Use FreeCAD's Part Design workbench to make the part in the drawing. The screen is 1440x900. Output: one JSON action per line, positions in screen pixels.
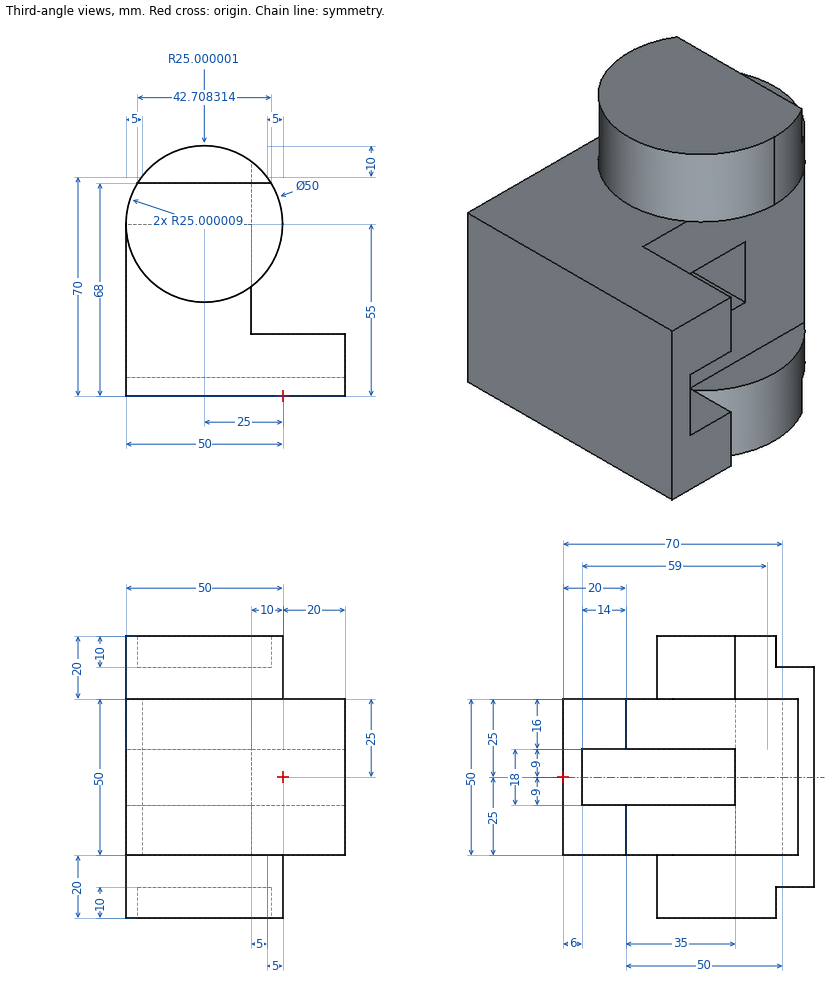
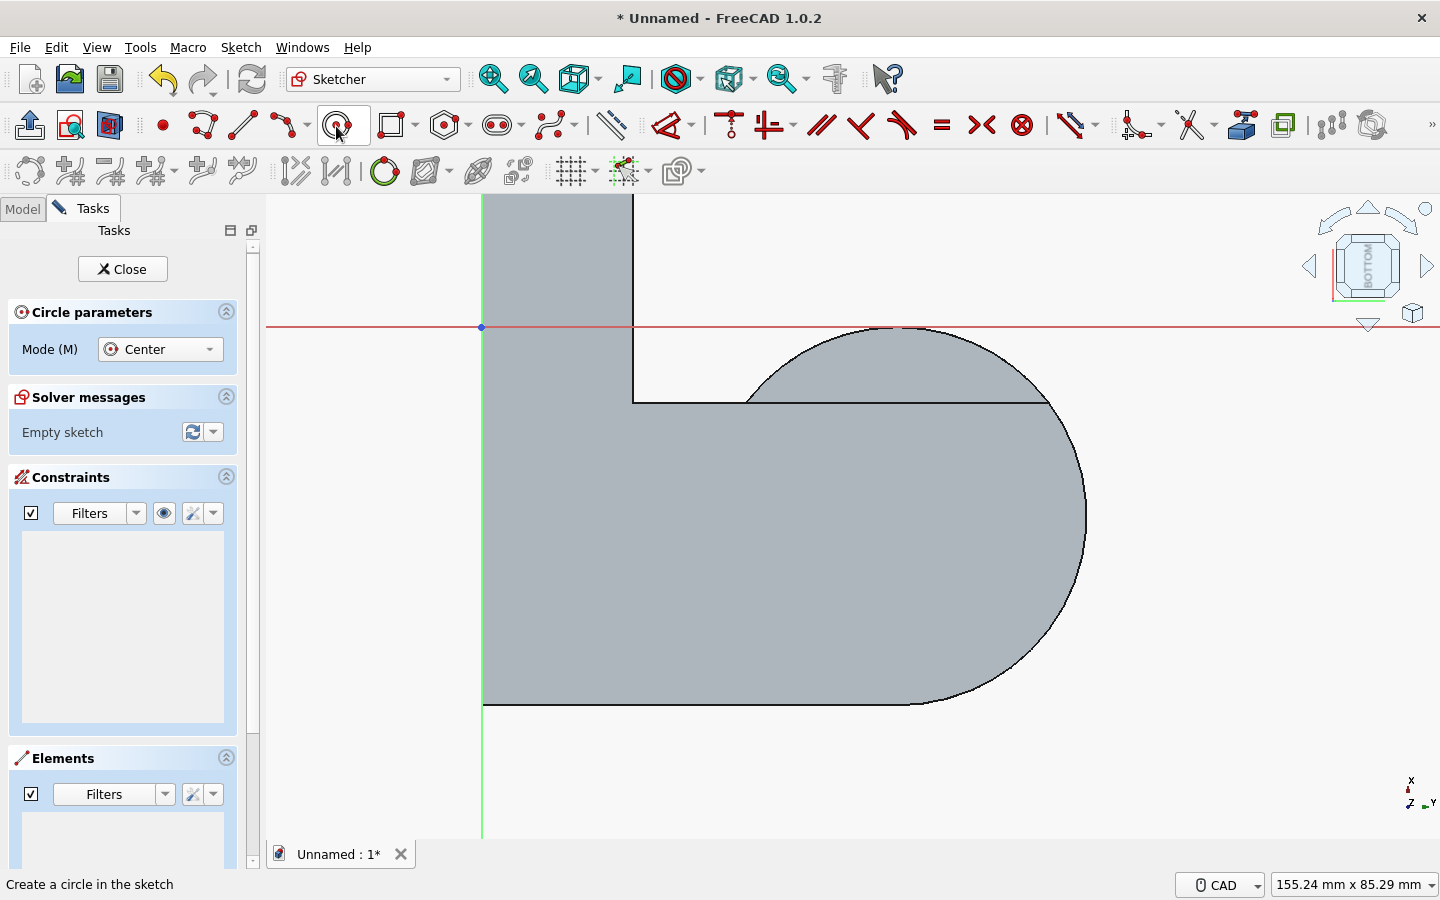
{"action": "left_click", "coordinate": [898, 516]}
{"action": "mouse_move", "coordinate": [1031, 383]}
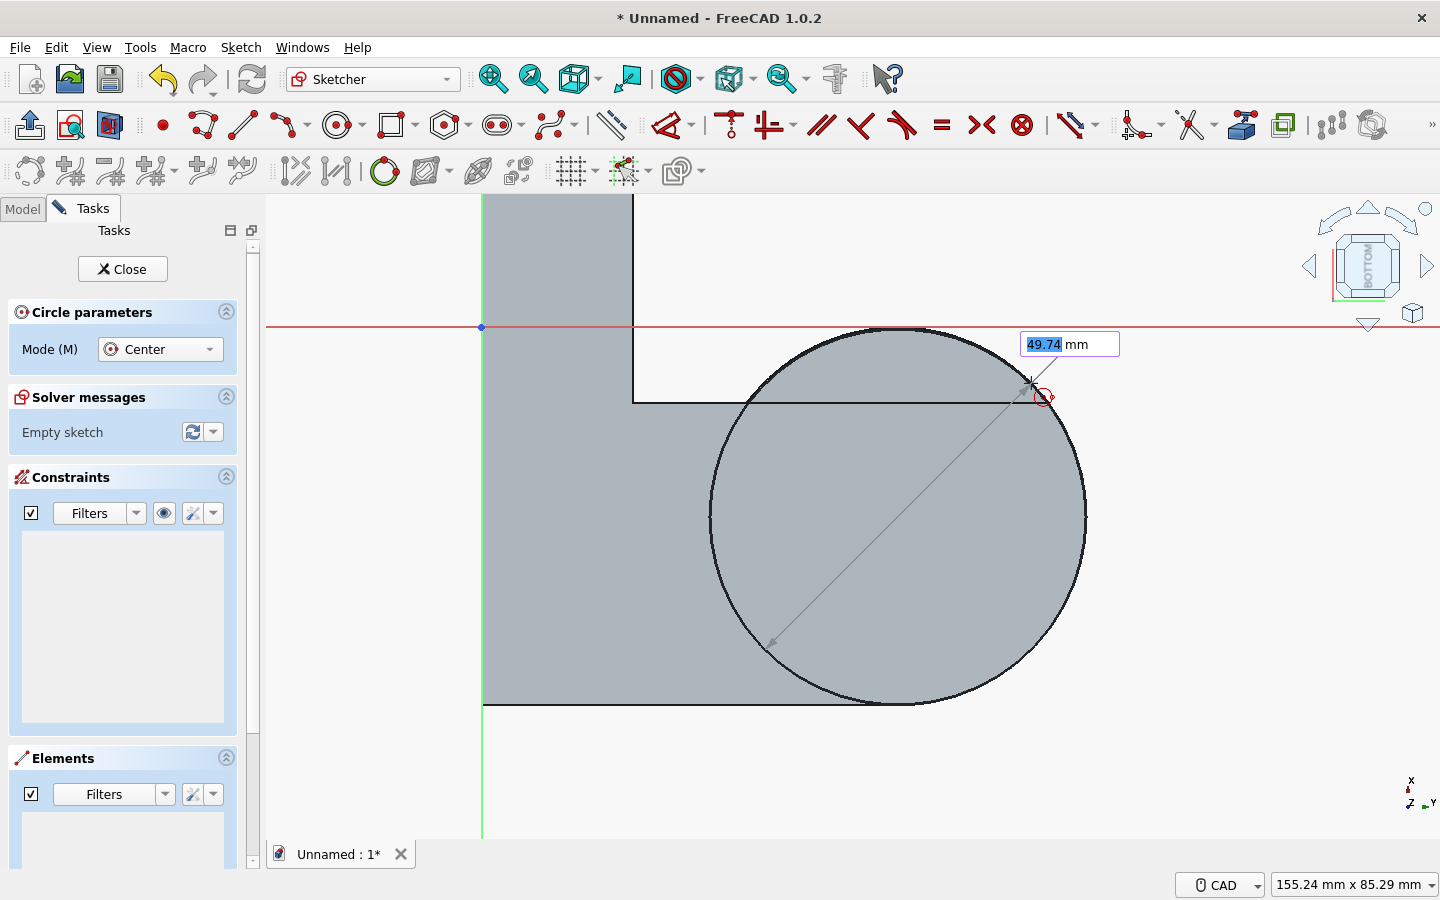
{"action": "type", "text": "50"}
{"action": "key", "text": "Return"}
{"action": "key", "text": "Escape"}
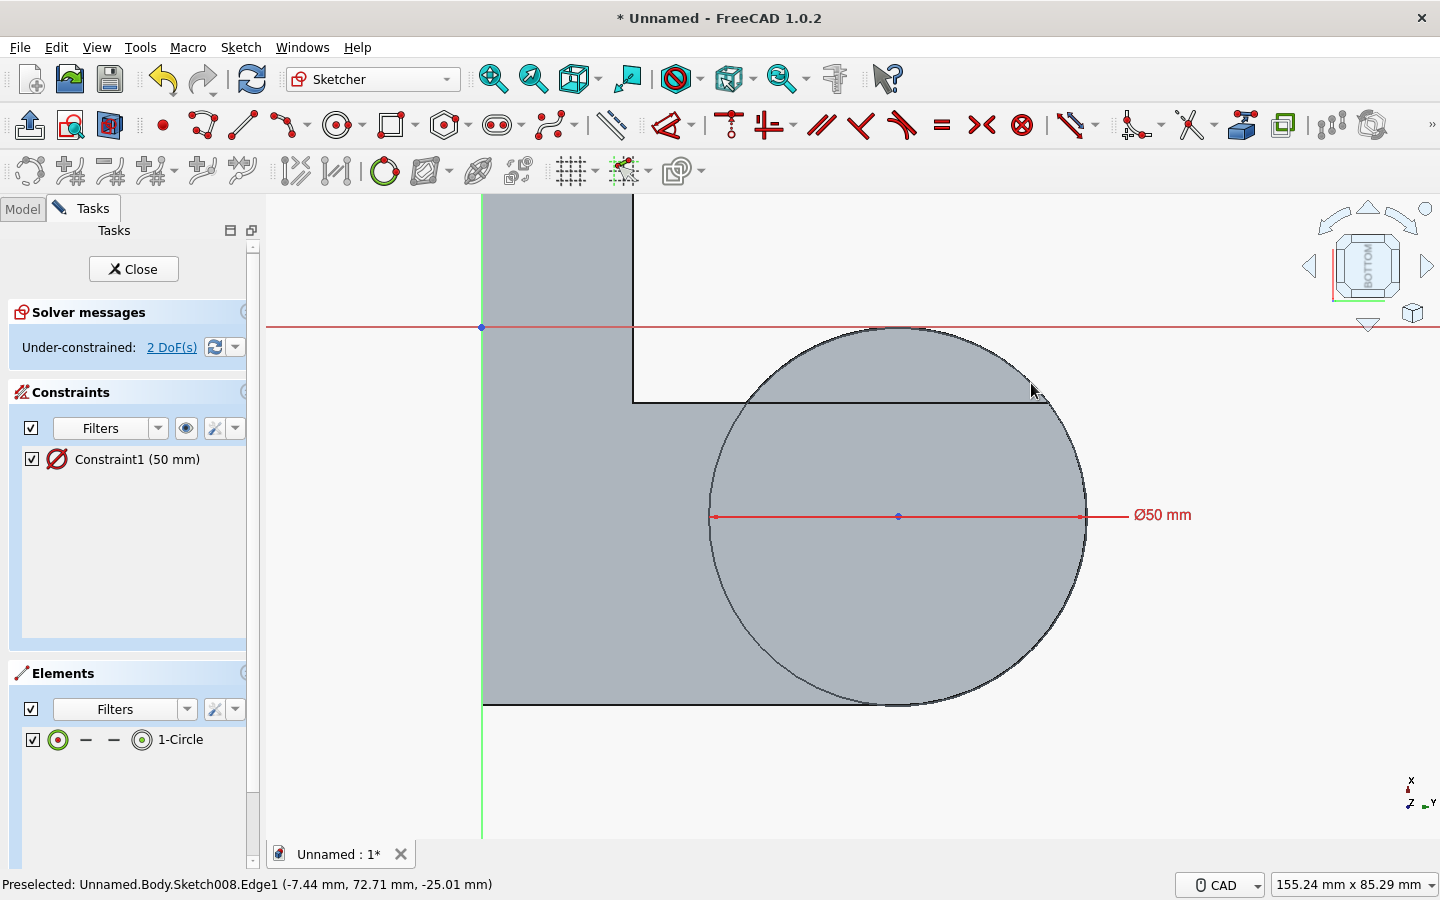
{"action": "key", "text": "d"}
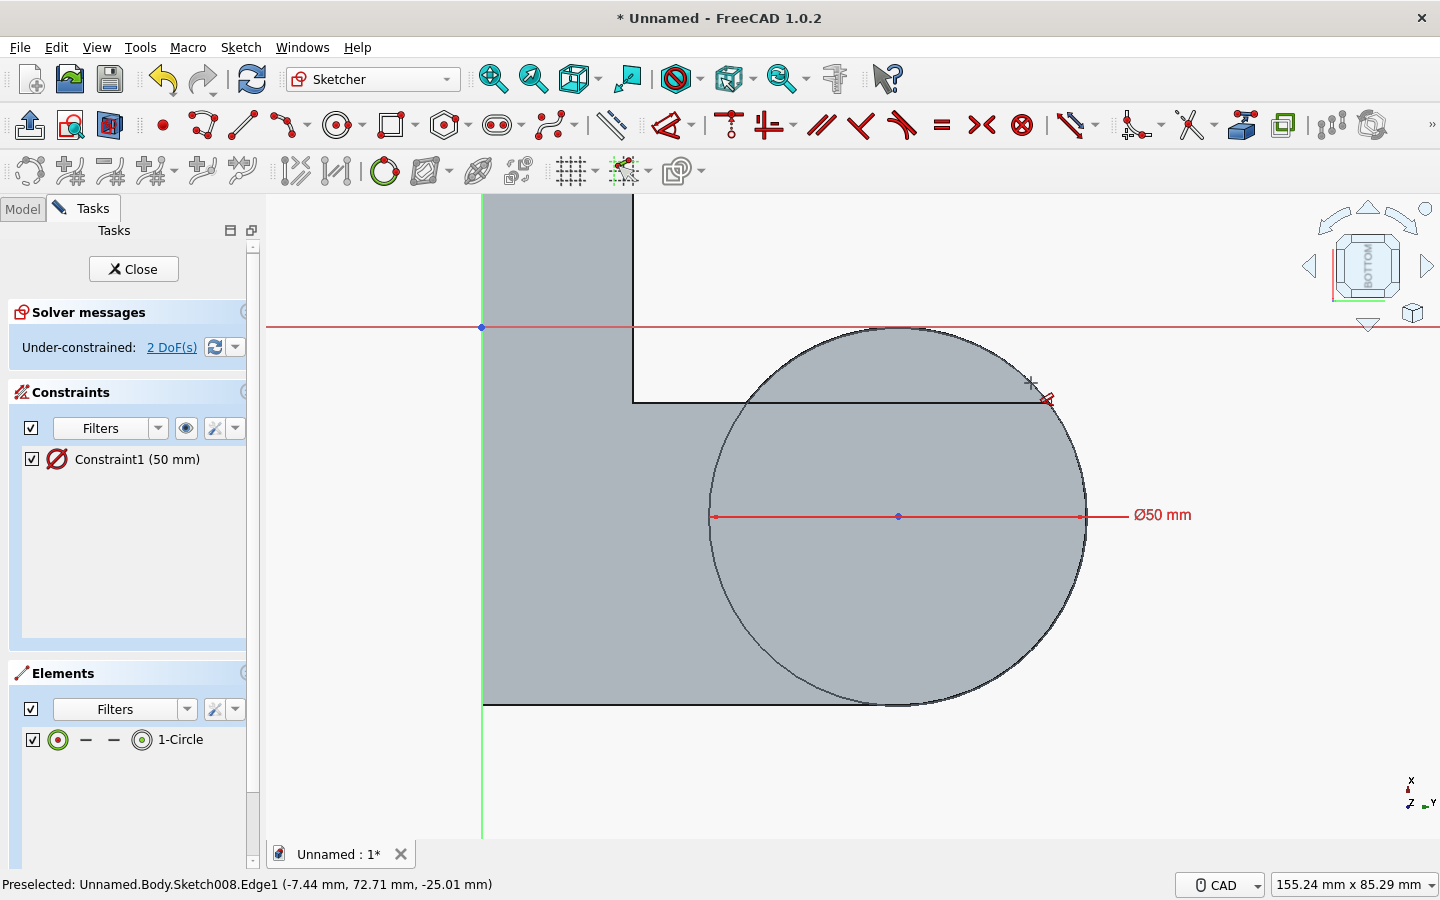
{"action": "left_click", "coordinate": [898, 517]}
{"action": "left_click", "coordinate": [690, 293]}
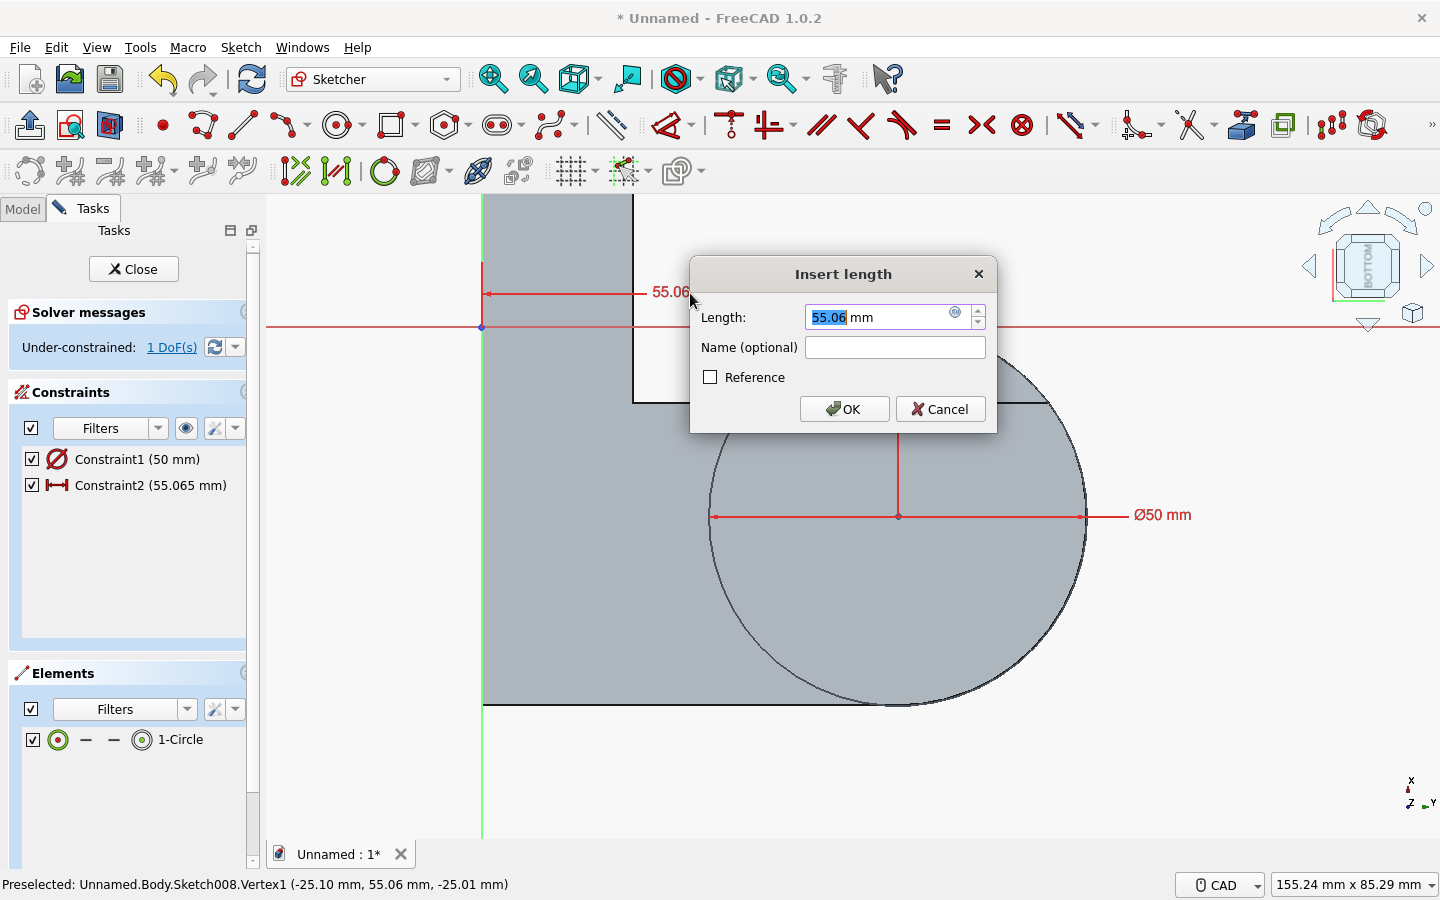
{"action": "type", "text": "55"}
{"action": "key", "text": "Return"}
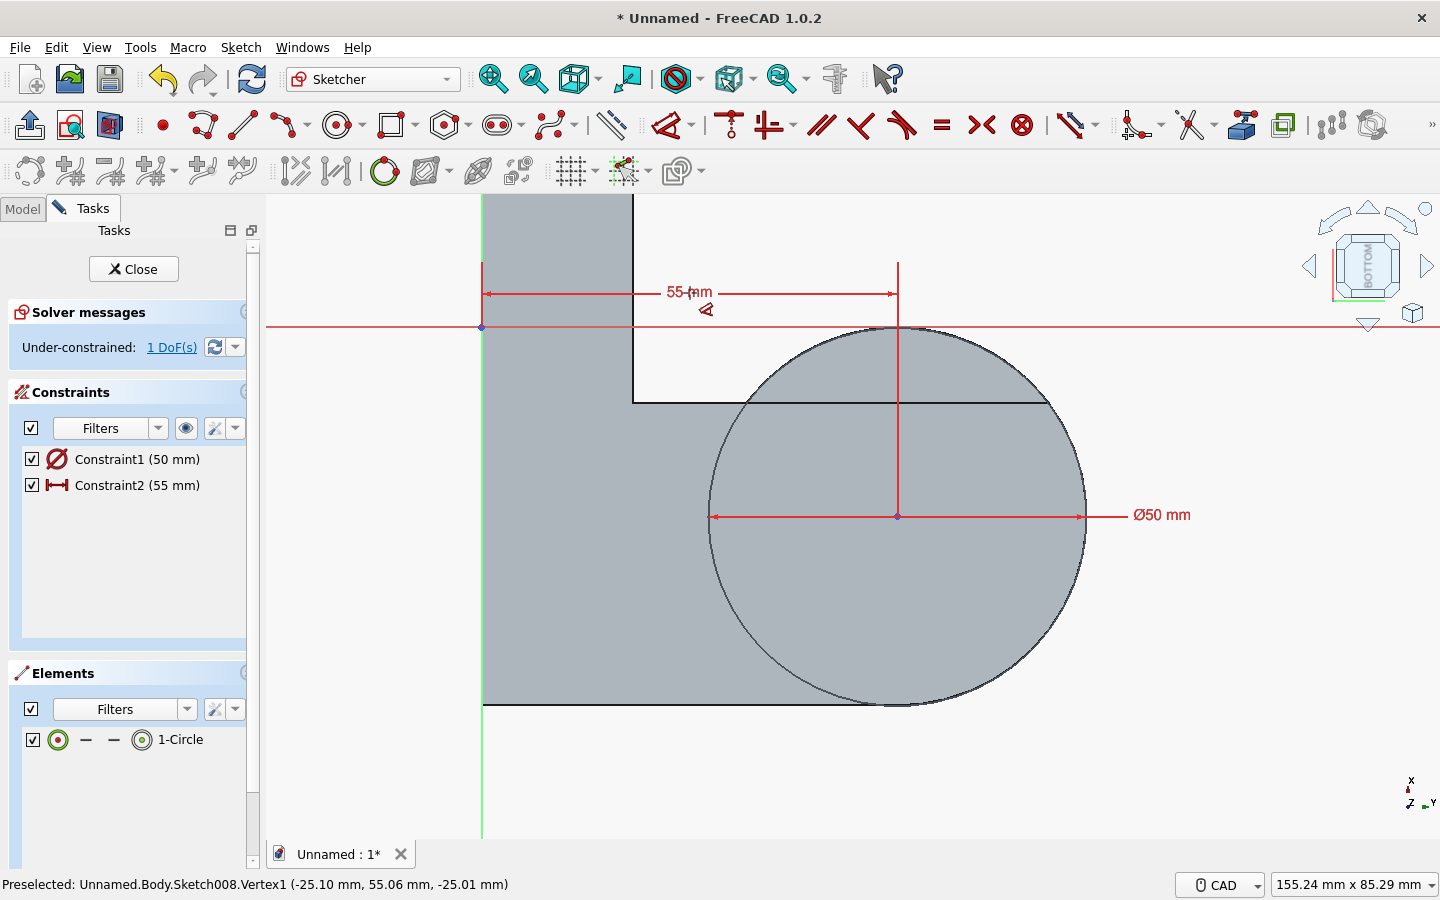
{"action": "left_click", "coordinate": [898, 517]}
{"action": "left_click", "coordinate": [448, 422]}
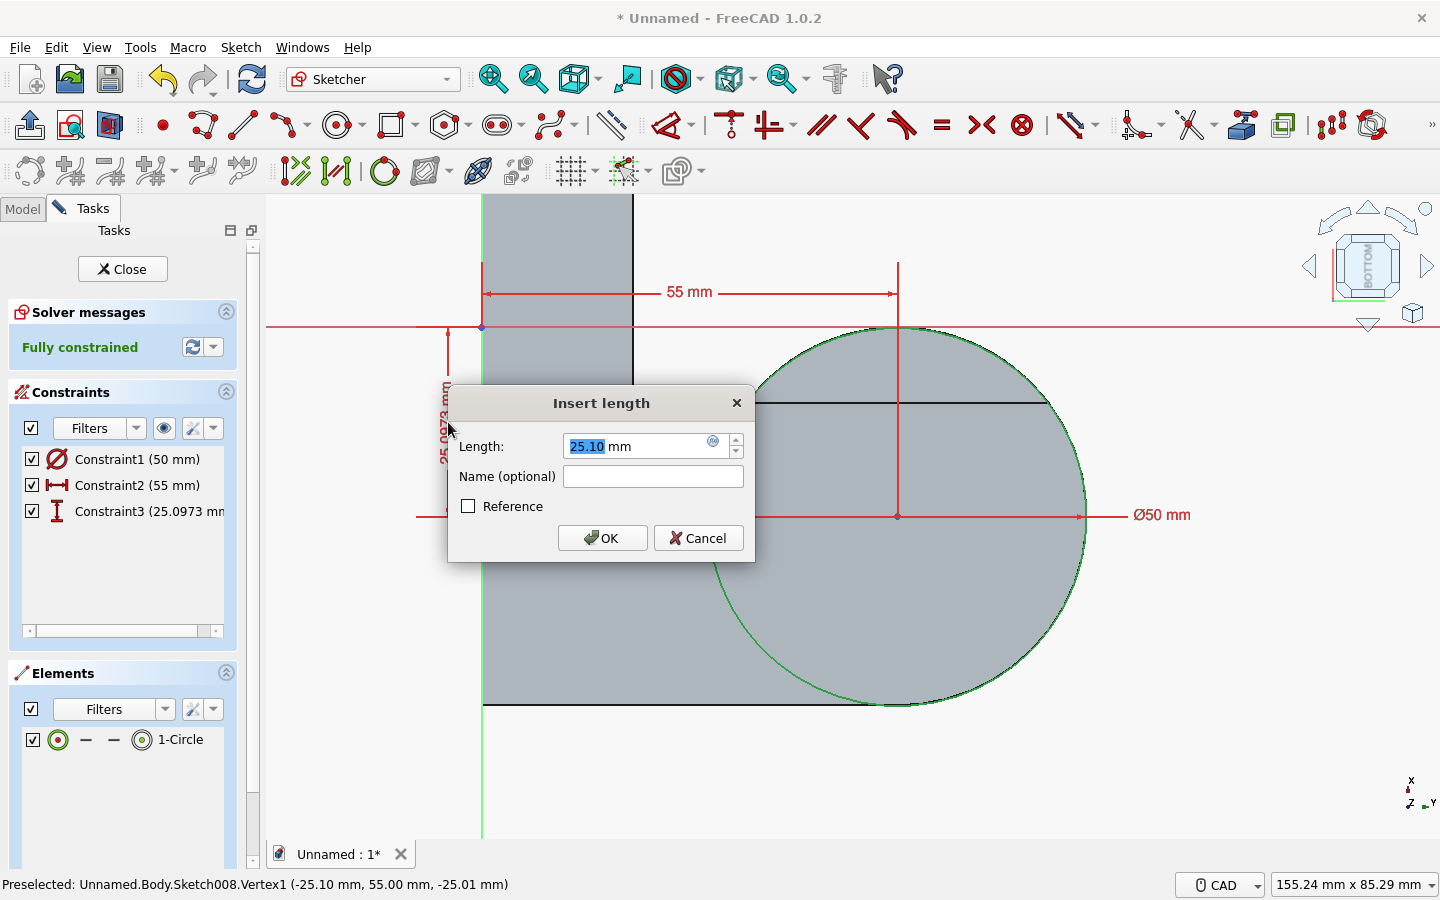
{"action": "type", "text": "25"}
{"action": "key", "text": "Return"}
{"action": "key", "text": "Escape"}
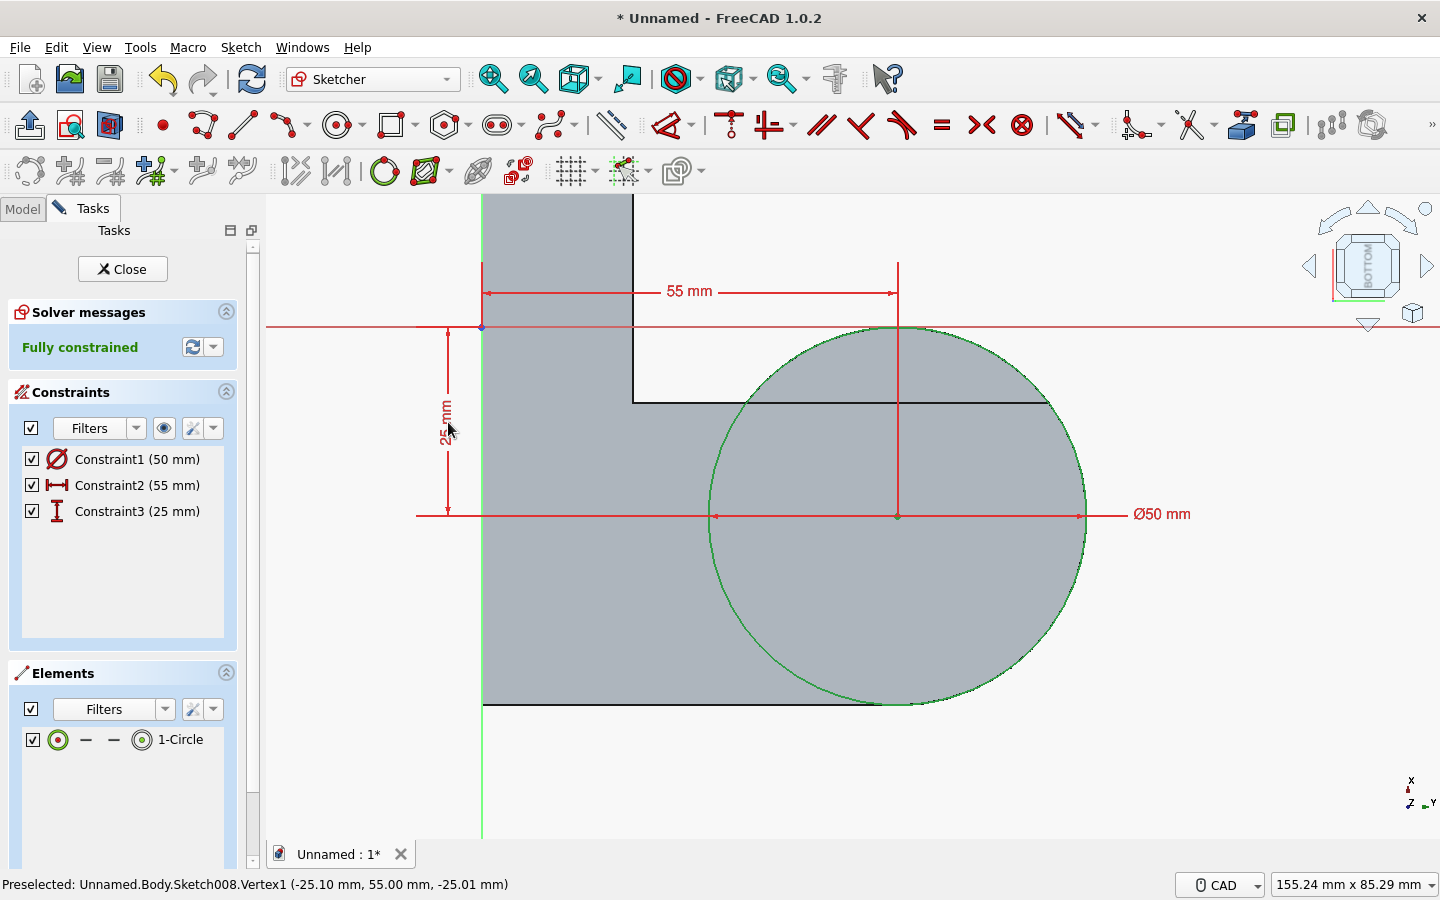
{"action": "left_click", "coordinate": [123, 269]}